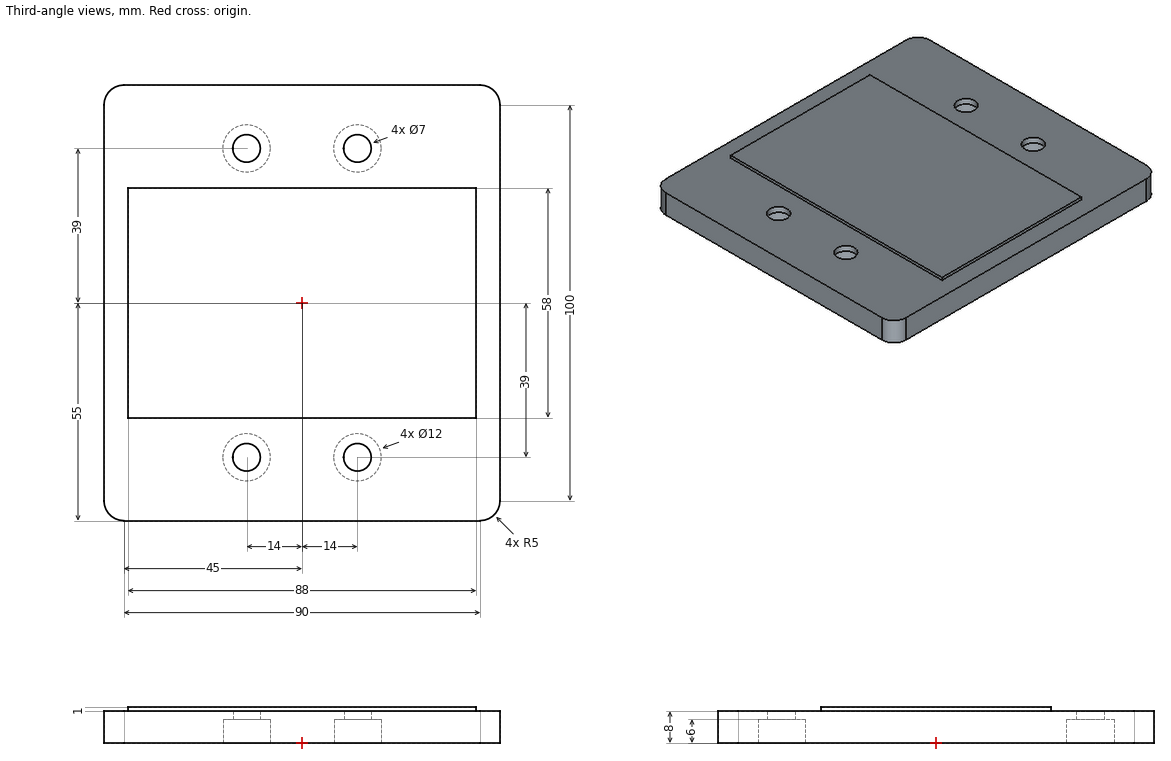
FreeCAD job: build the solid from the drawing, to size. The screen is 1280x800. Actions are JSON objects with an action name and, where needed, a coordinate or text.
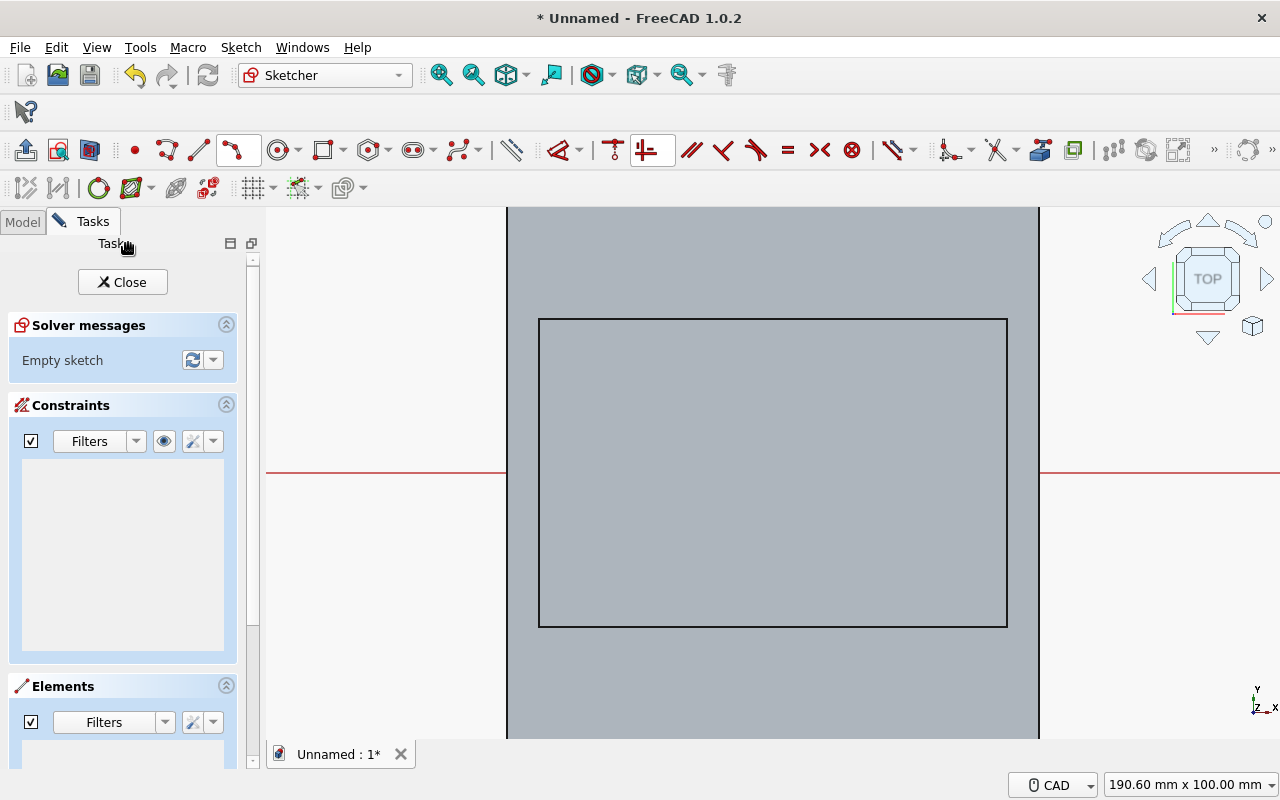
{"action": "left_click", "coordinate": [90, 150]}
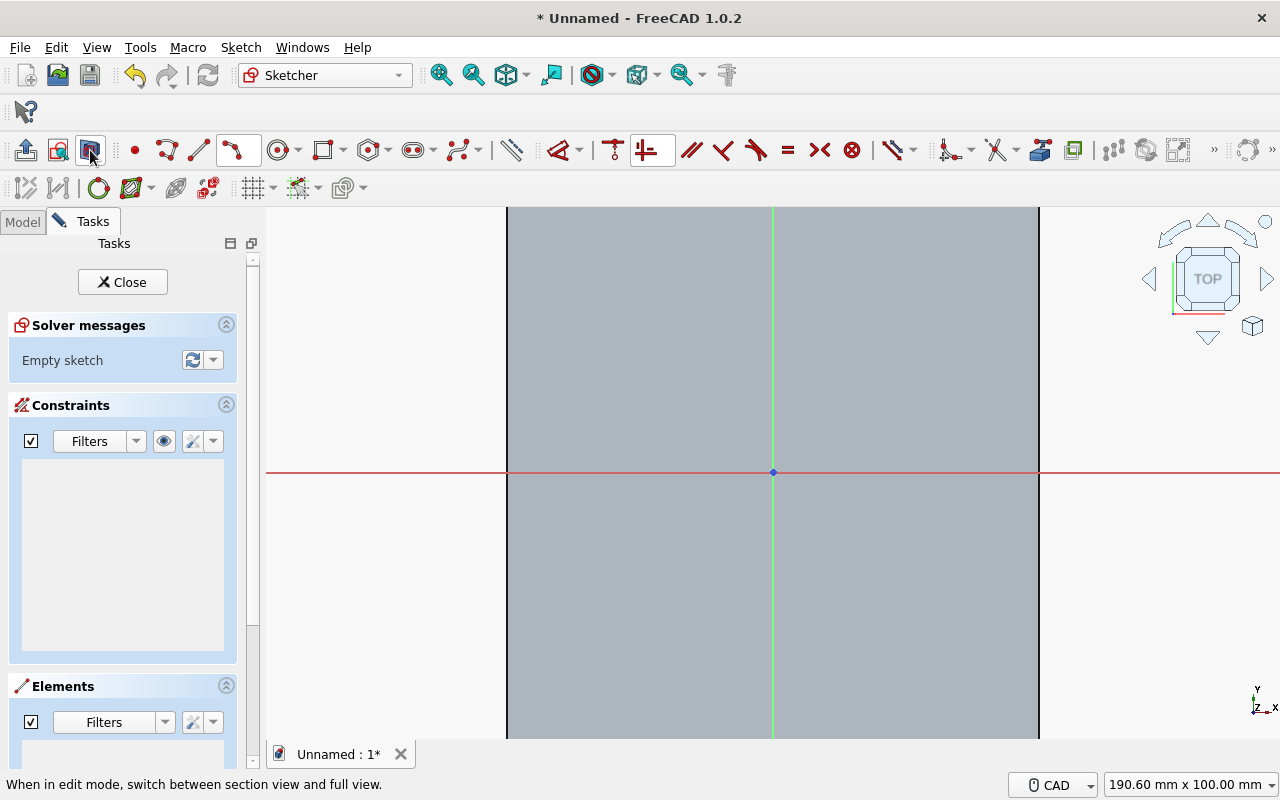
{"action": "scroll", "coordinate": [565, 473], "scroll_direction": "down", "scroll_amount": 2}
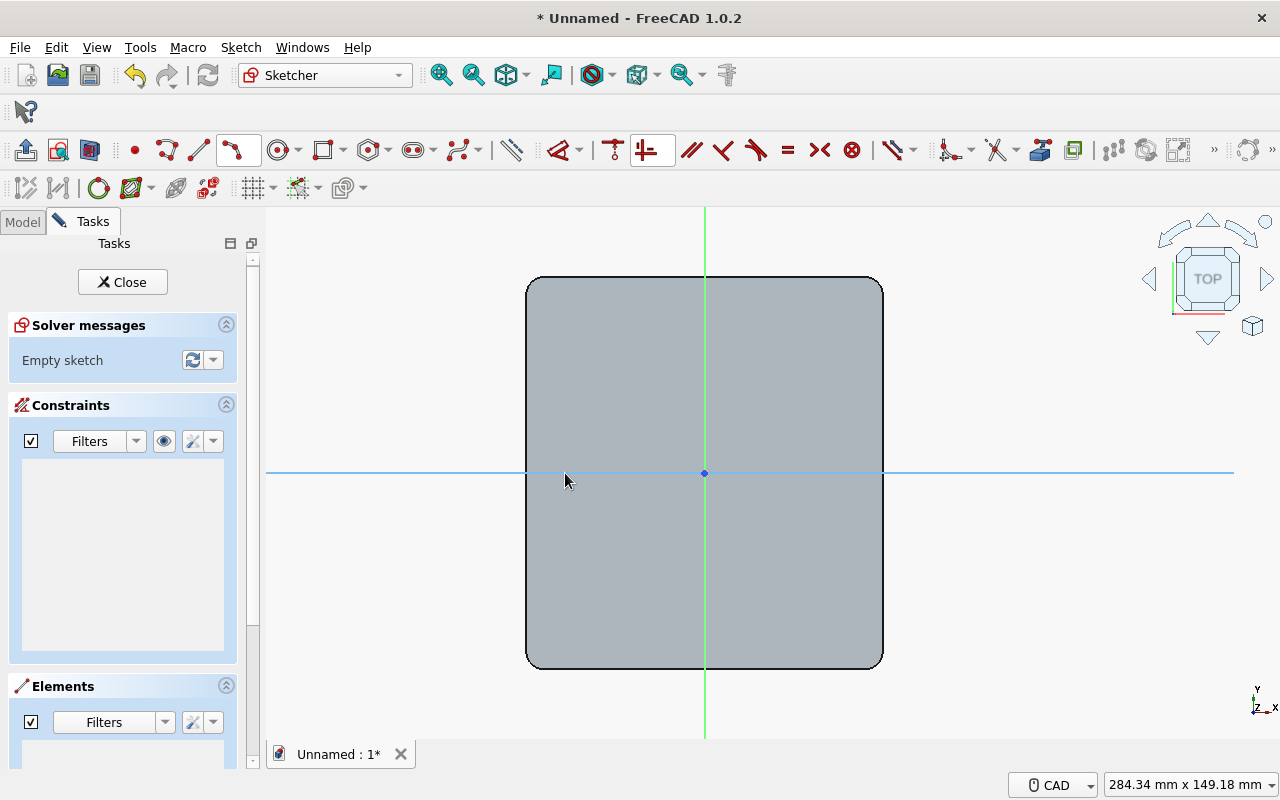
{"action": "left_click", "coordinate": [278, 150]}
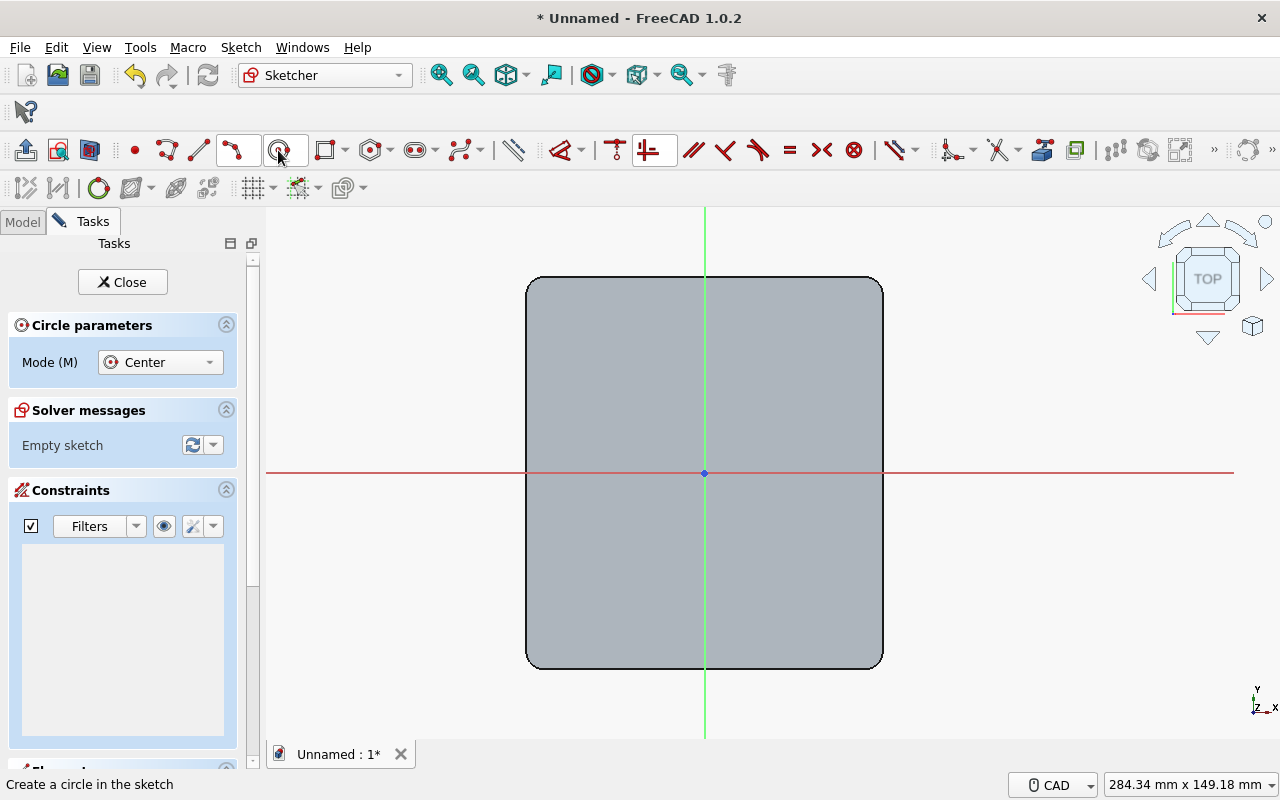
{"action": "left_click", "coordinate": [754, 612]}
{"action": "mouse_move", "coordinate": [770, 597]}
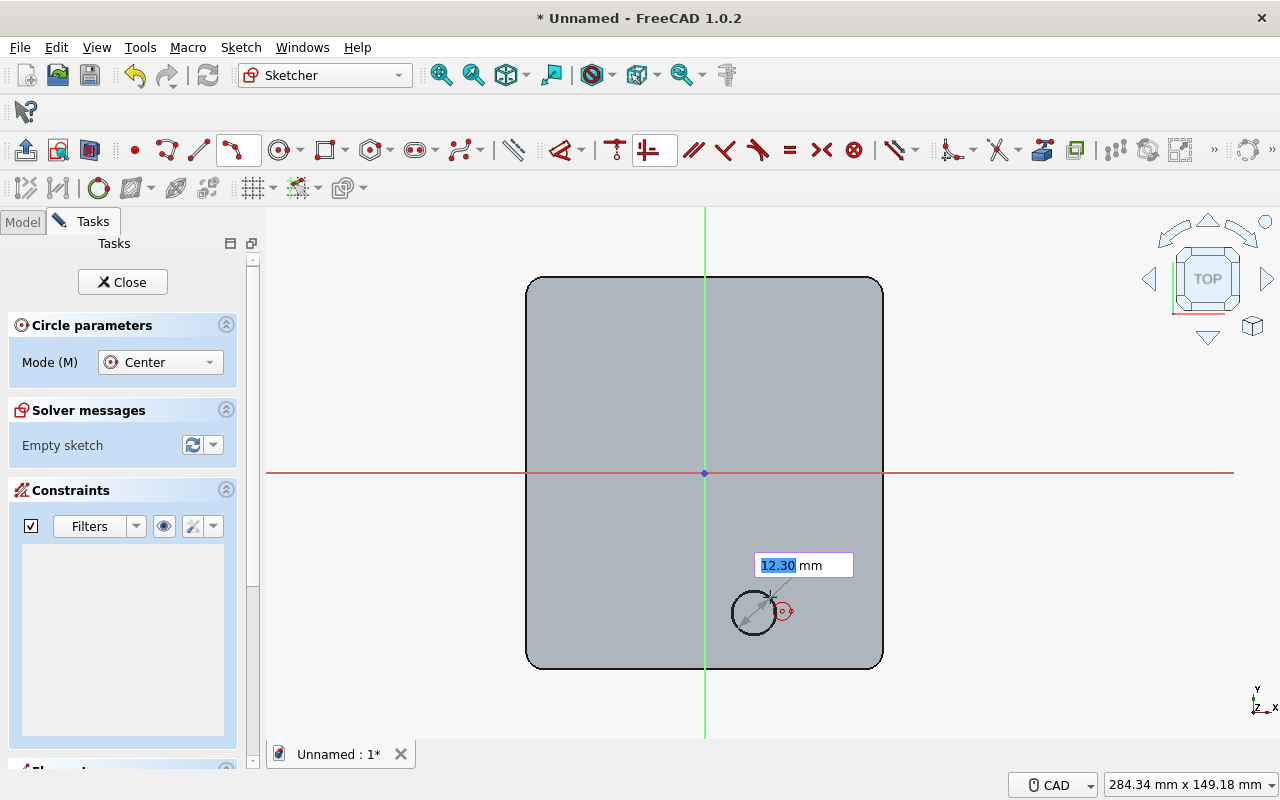
{"action": "type", "text": "12"}
{"action": "key", "text": "Return"}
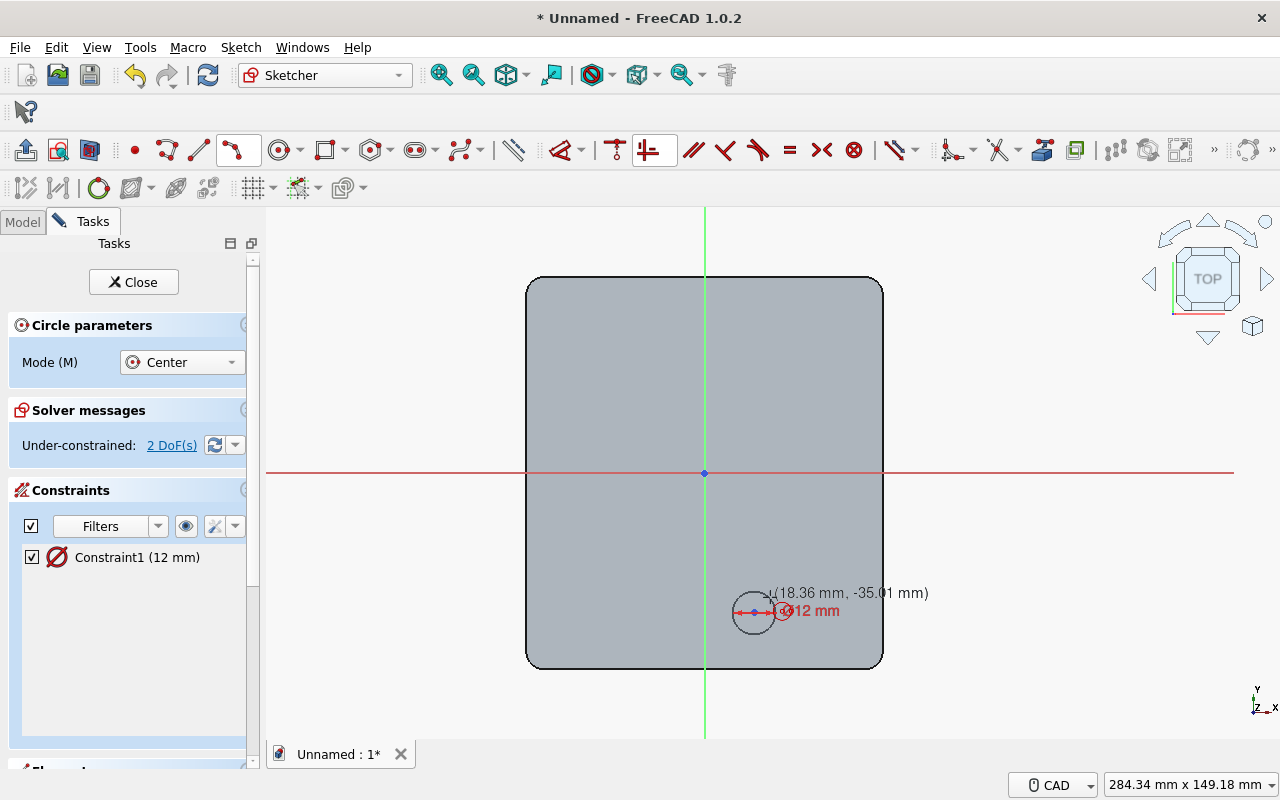
{"action": "left_click", "coordinate": [655, 612]}
{"action": "mouse_move", "coordinate": [670, 597]}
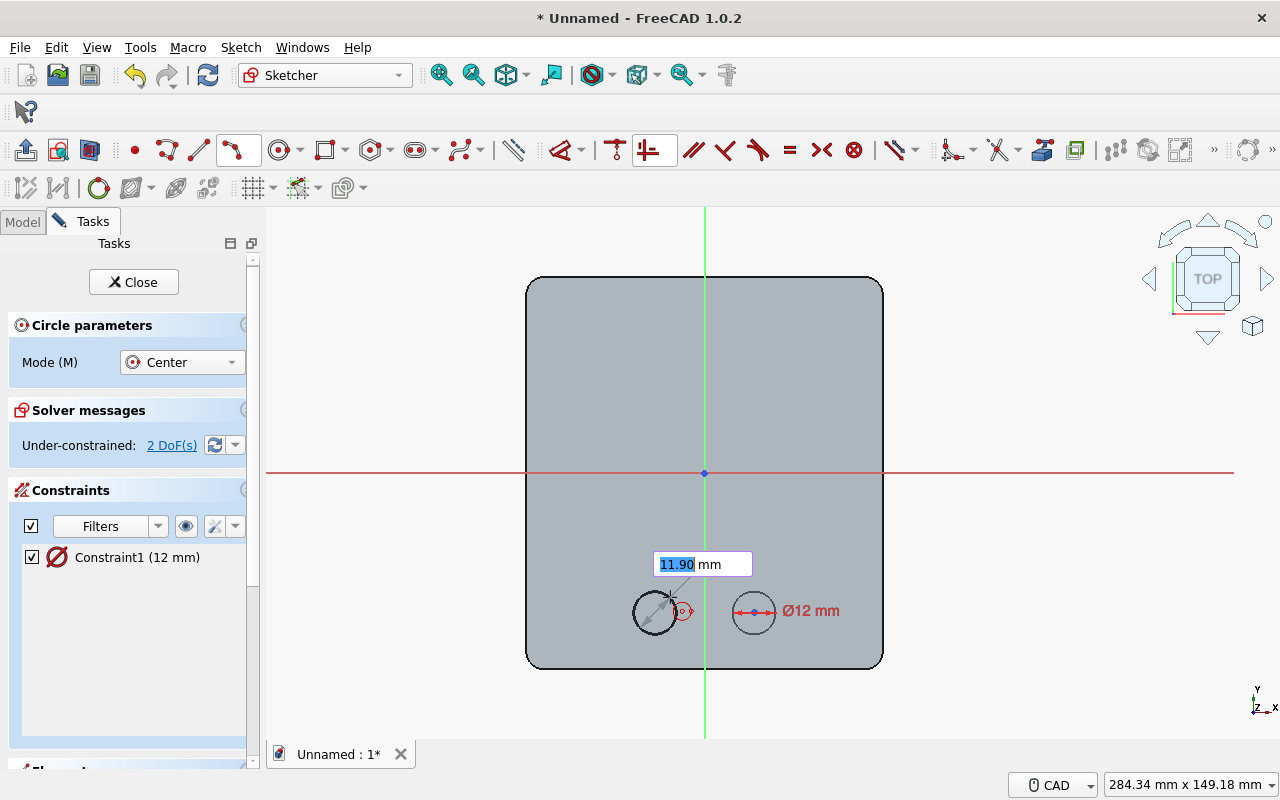
{"action": "type", "text": "12"}
{"action": "key", "text": "Return"}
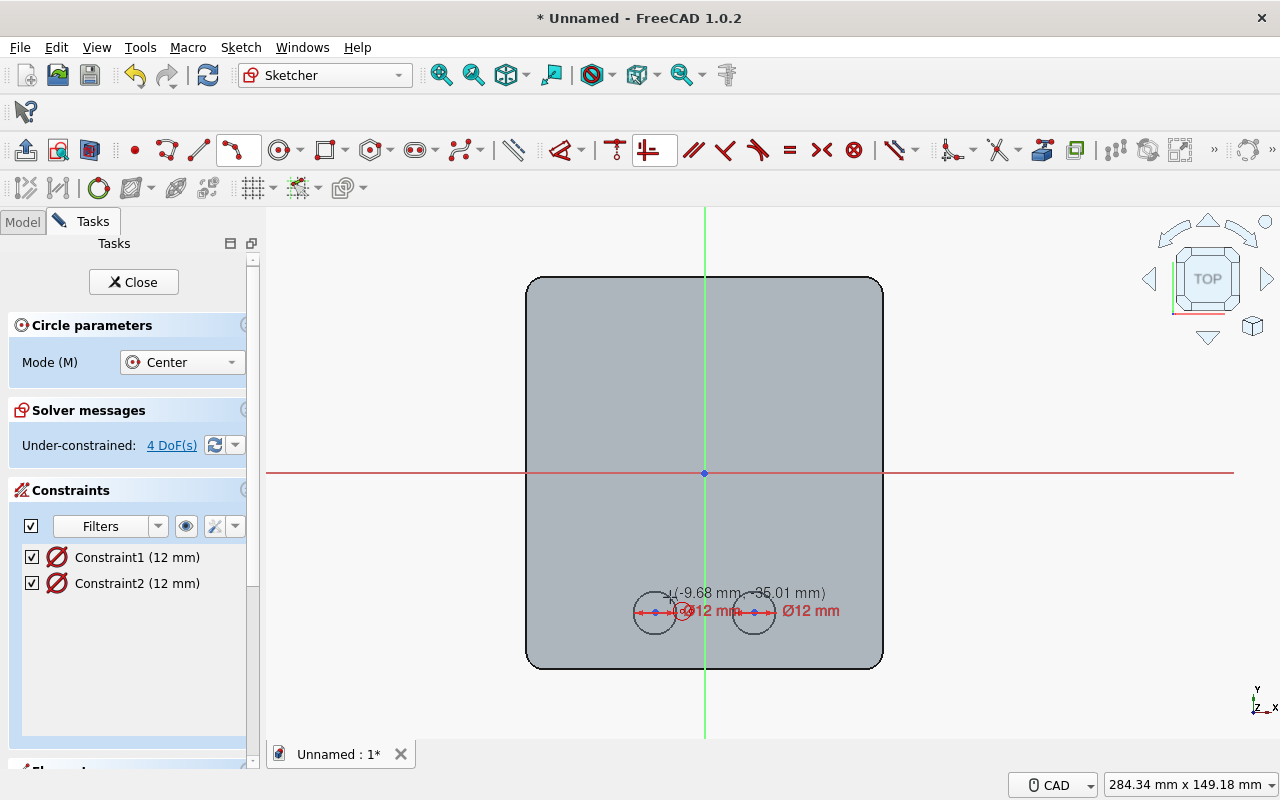
{"action": "left_click", "coordinate": [655, 334]}
{"action": "mouse_move", "coordinate": [670, 319]}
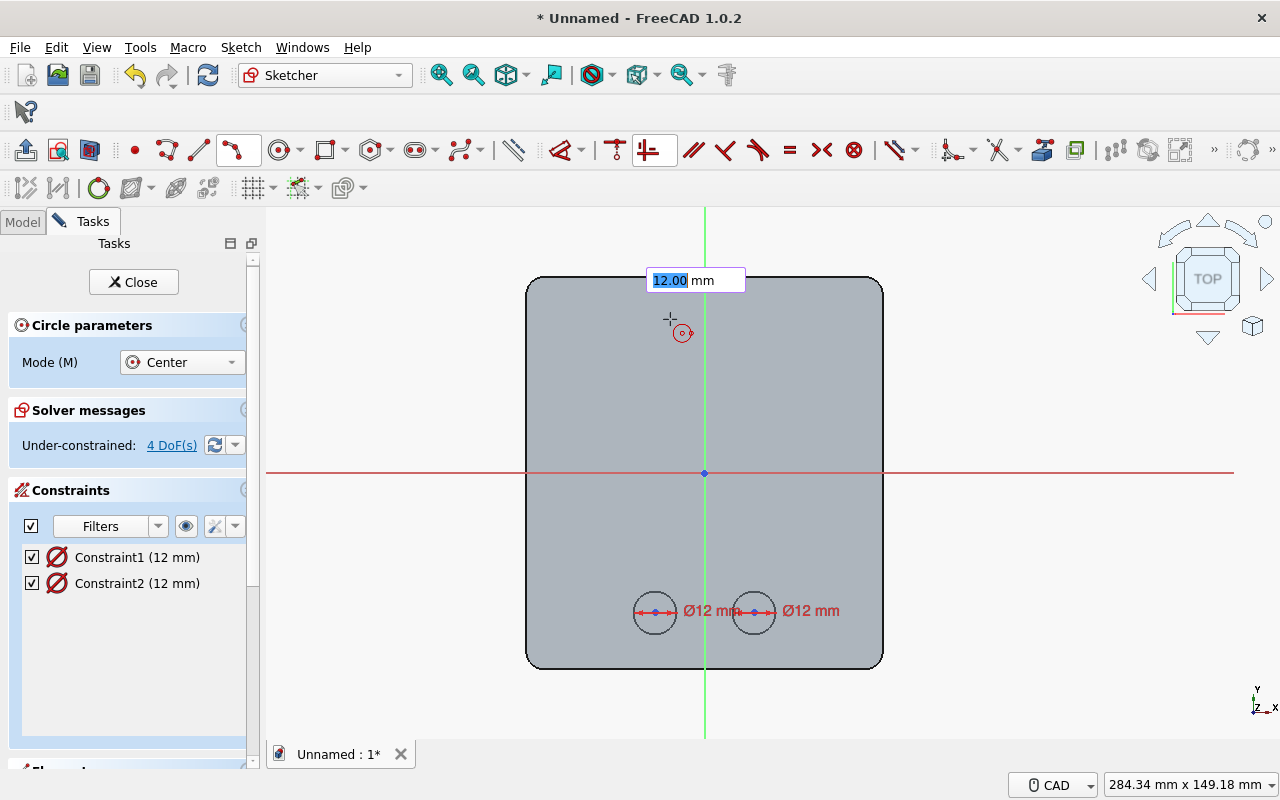
{"action": "type", "text": "12"}
{"action": "key", "text": "Return"}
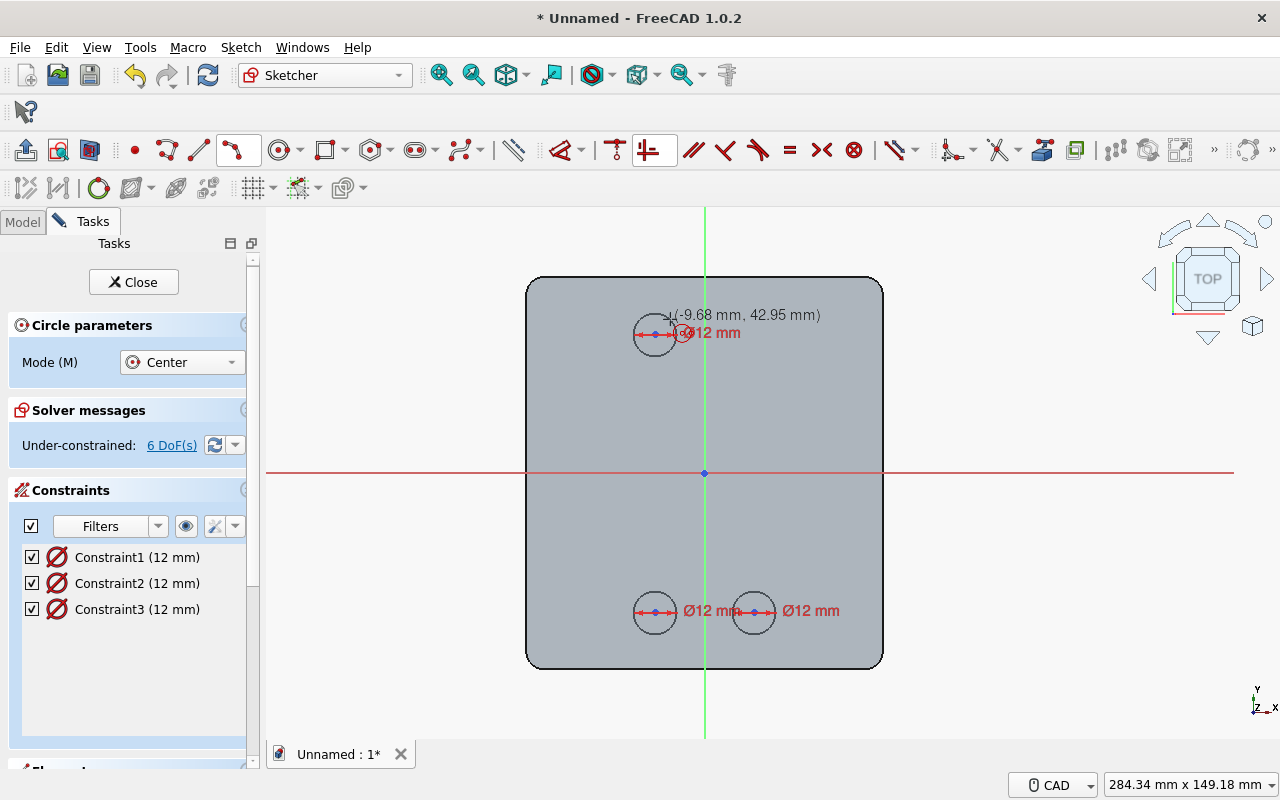
{"action": "left_click", "coordinate": [754, 334]}
{"action": "mouse_move", "coordinate": [770, 319]}